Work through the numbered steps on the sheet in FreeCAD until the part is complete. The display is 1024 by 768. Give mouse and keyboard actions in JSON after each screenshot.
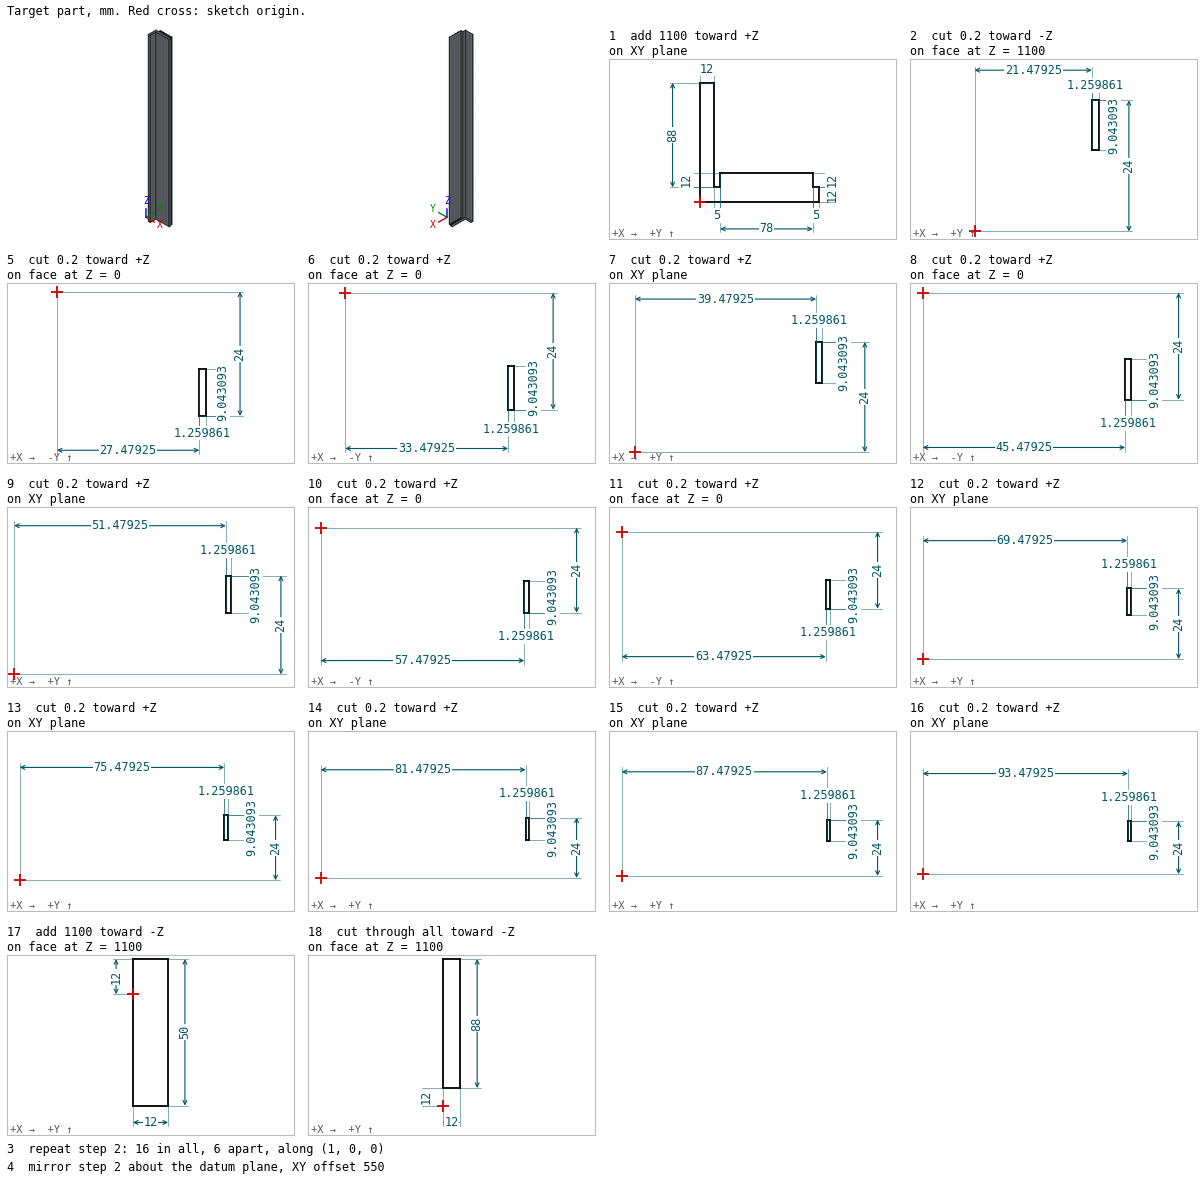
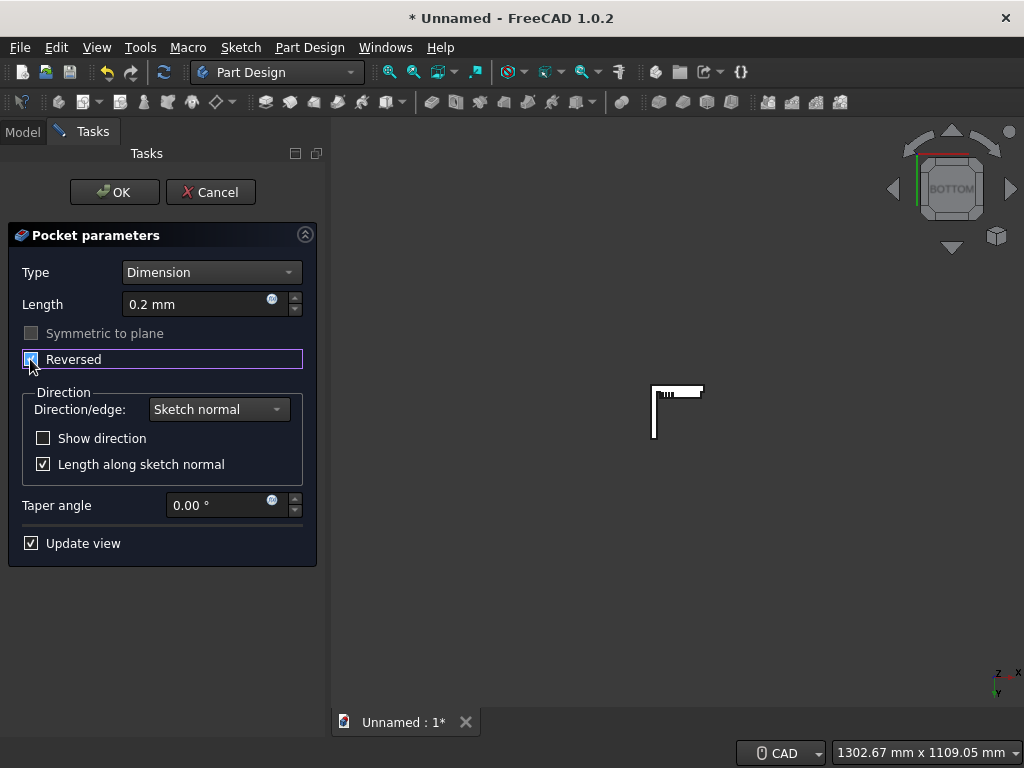
{"action": "left_click", "coordinate": [115, 192]}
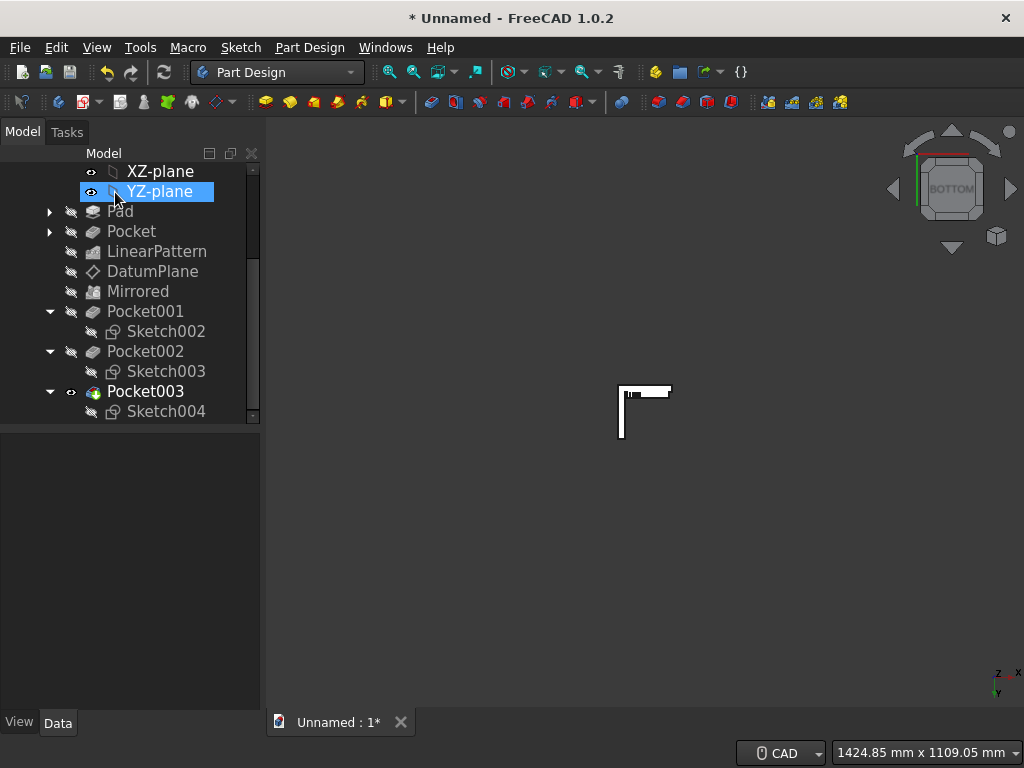
{"action": "left_click", "coordinate": [390, 72]}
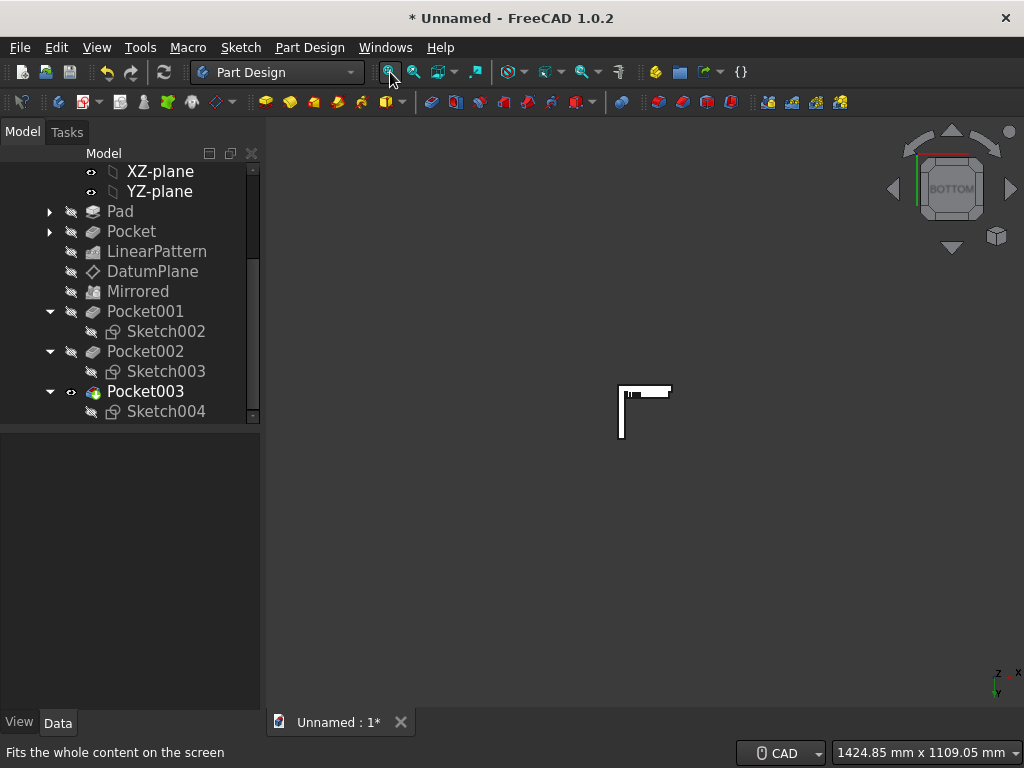
{"action": "left_click", "coordinate": [660, 388]}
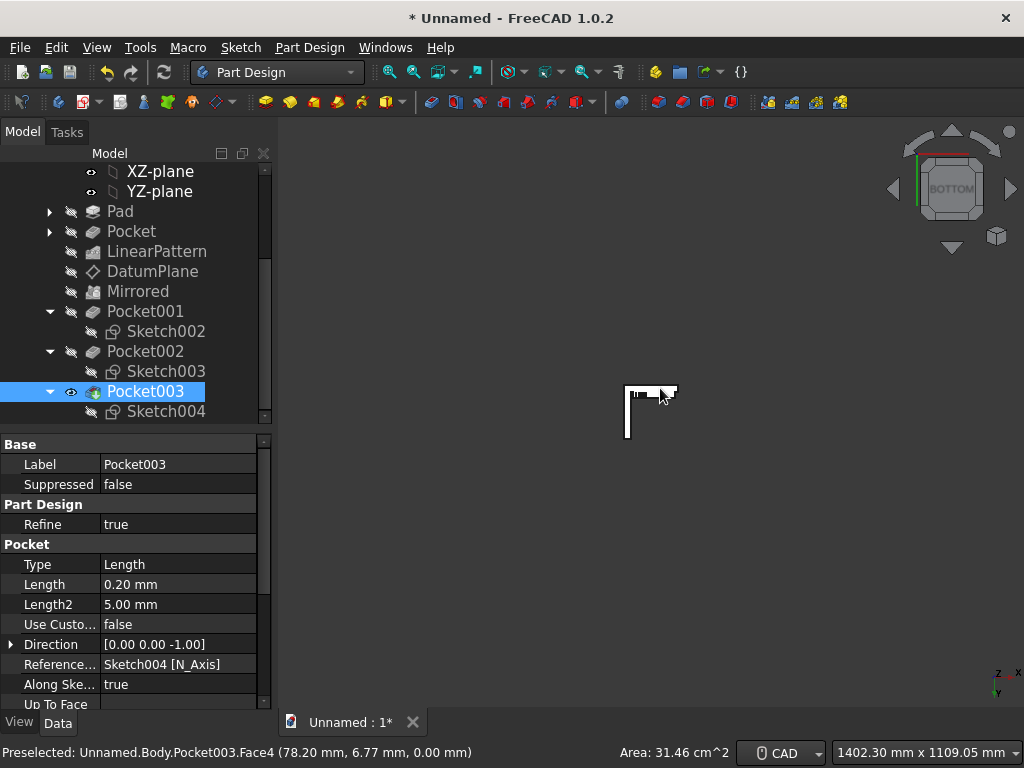
{"action": "left_click", "coordinate": [84, 102]}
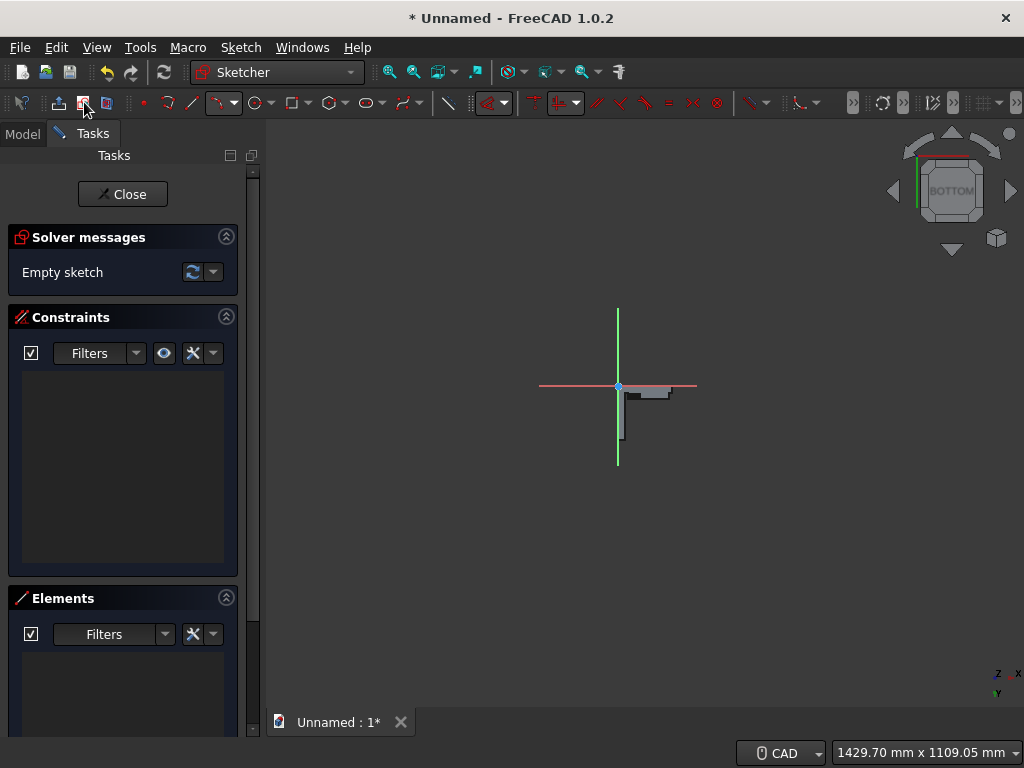
{"action": "scroll", "coordinate": [646, 396], "scroll_direction": "up", "scroll_amount": 15}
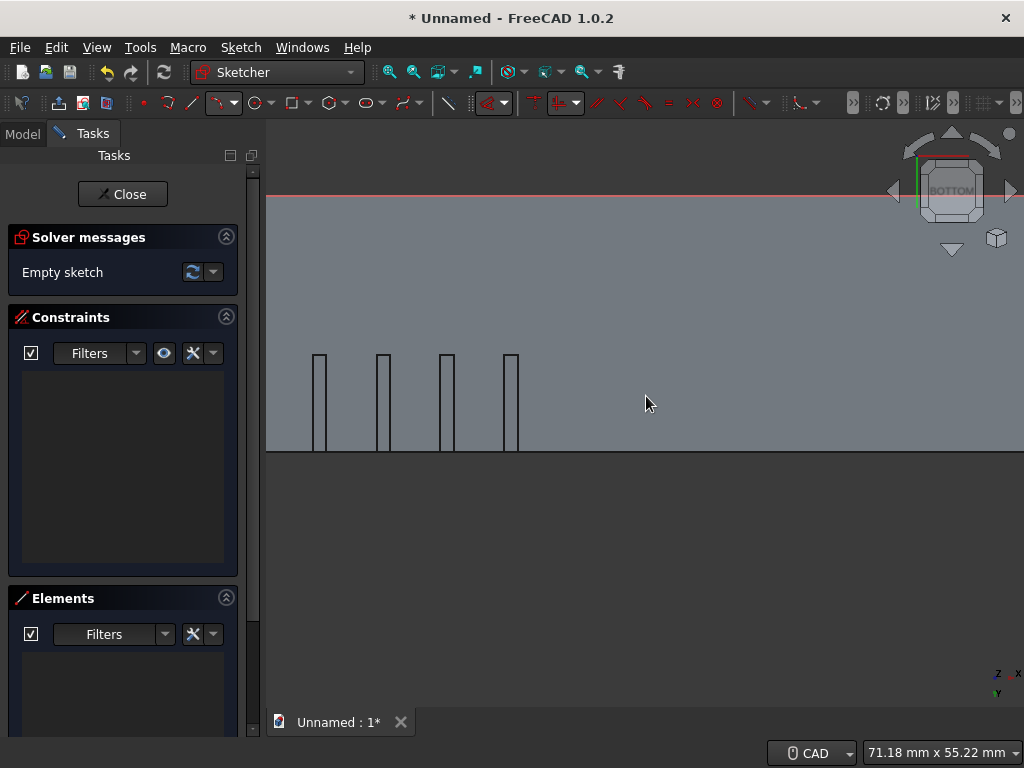
{"action": "scroll", "coordinate": [574, 400], "scroll_direction": "up", "scroll_amount": 7}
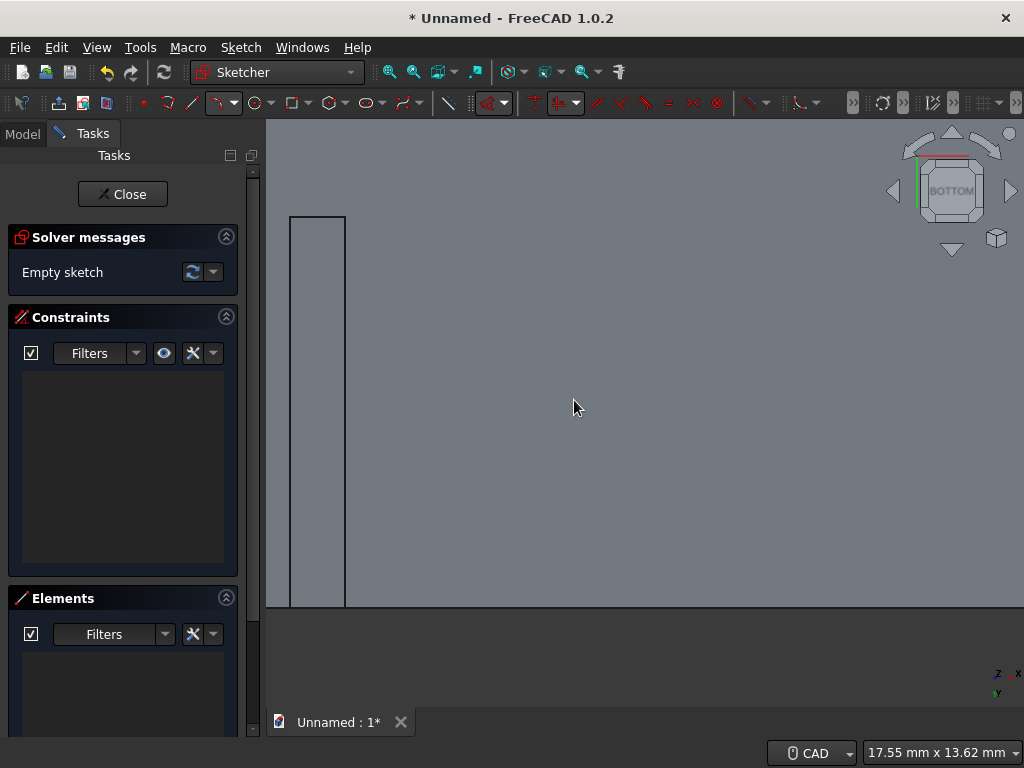
{"action": "left_click", "coordinate": [292, 104]}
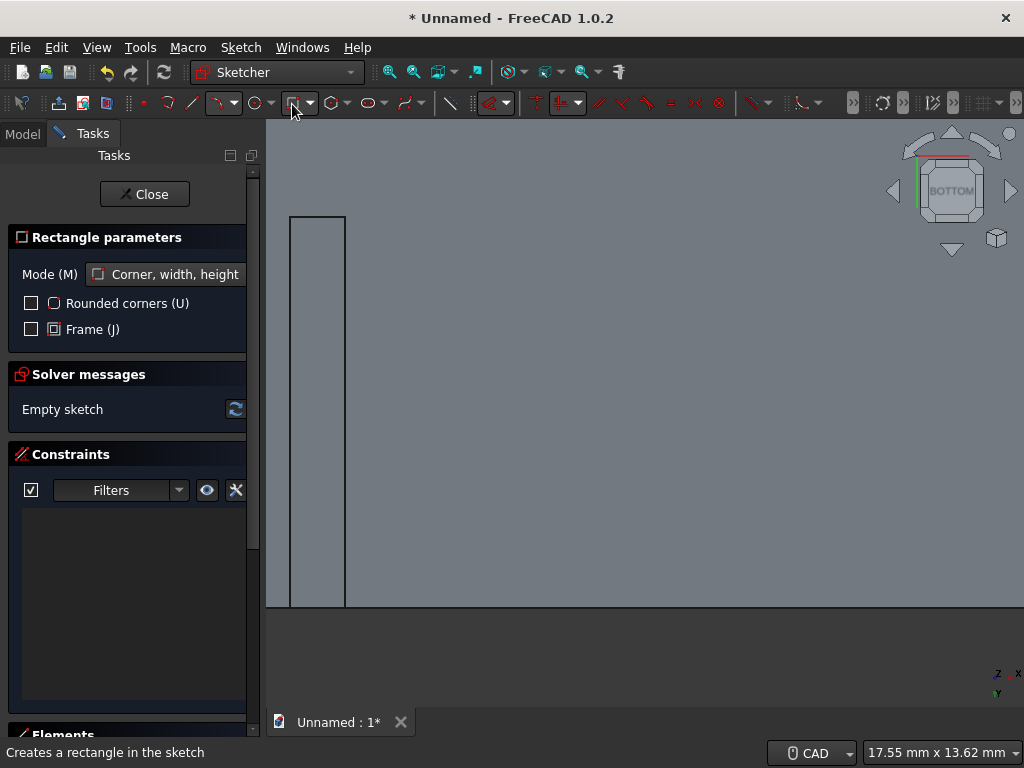
{"action": "left_click", "coordinate": [549, 217]}
{"action": "mouse_move", "coordinate": [604, 608]}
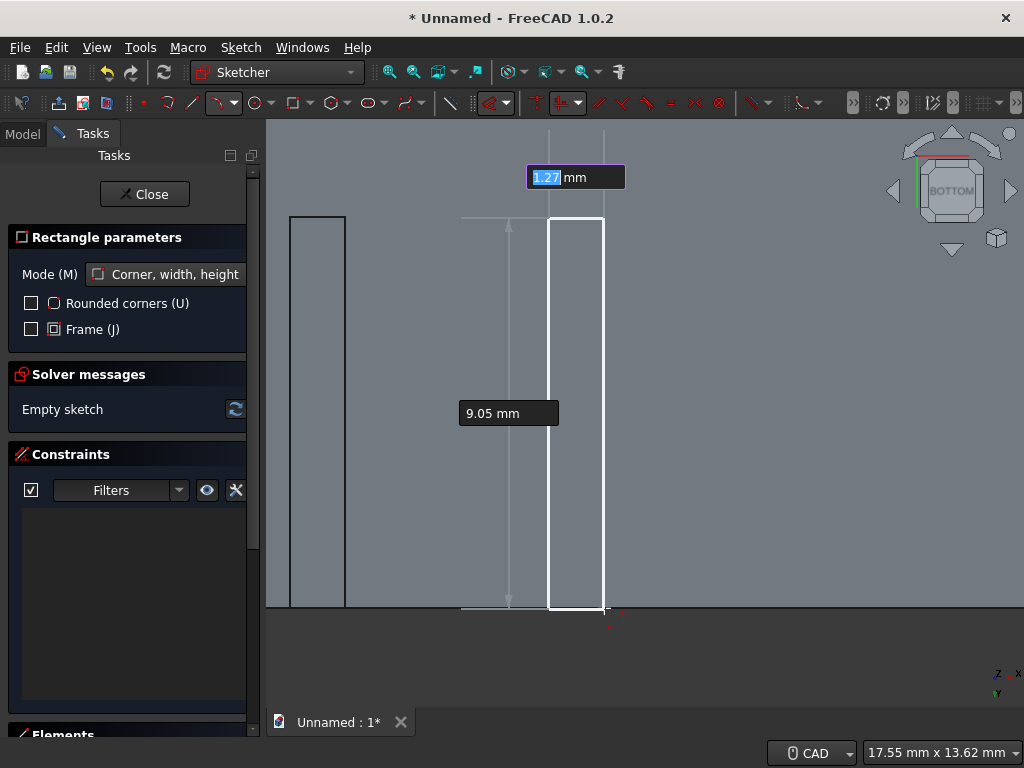
{"action": "type", "text": "1.259861"}
{"action": "key", "text": "Tab"}
{"action": "type", "text": "9.043093"}
{"action": "key", "text": "Return"}
{"action": "key", "text": "Escape"}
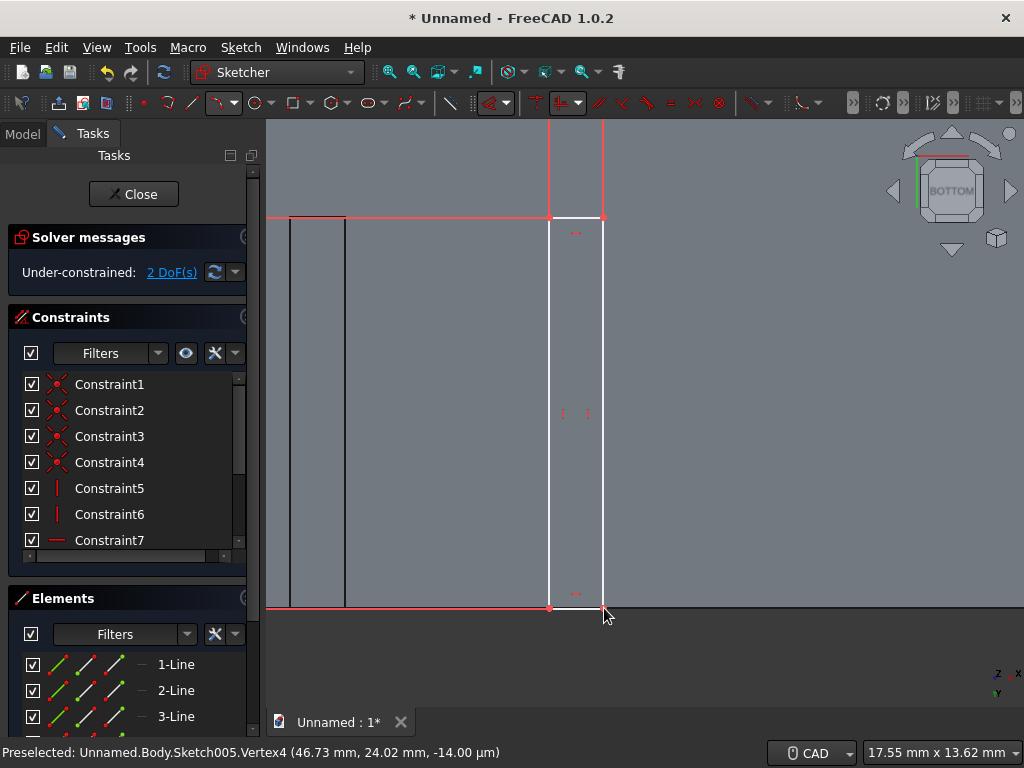
{"action": "left_click", "coordinate": [549, 609]}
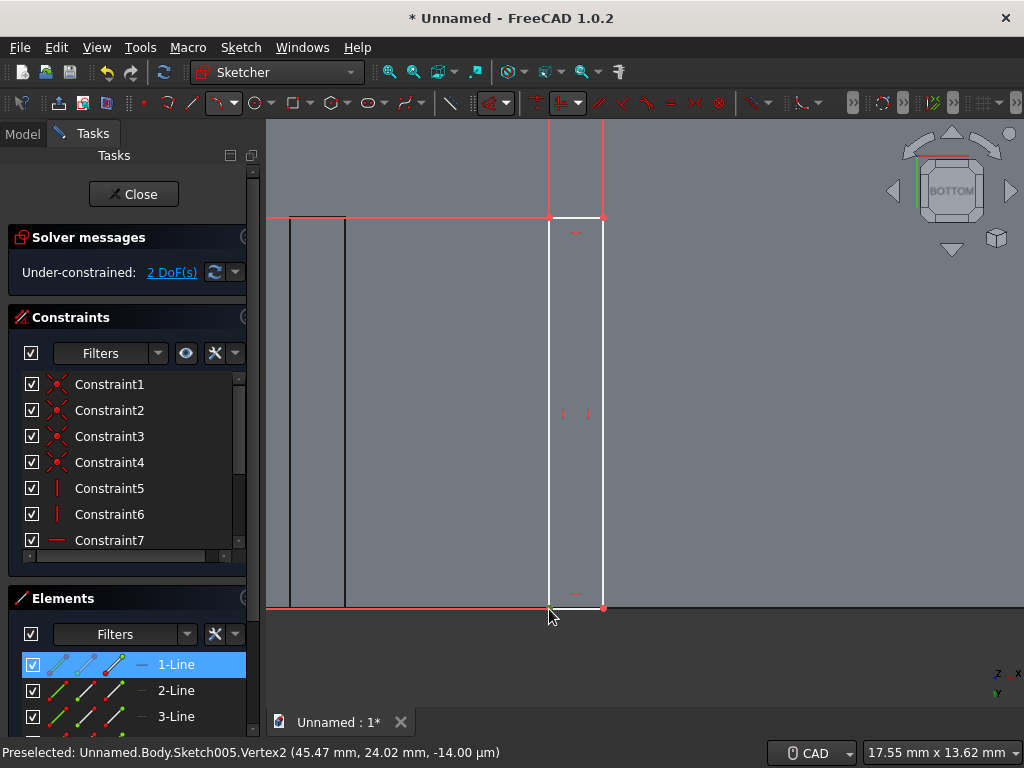
{"action": "left_click", "coordinate": [508, 104]}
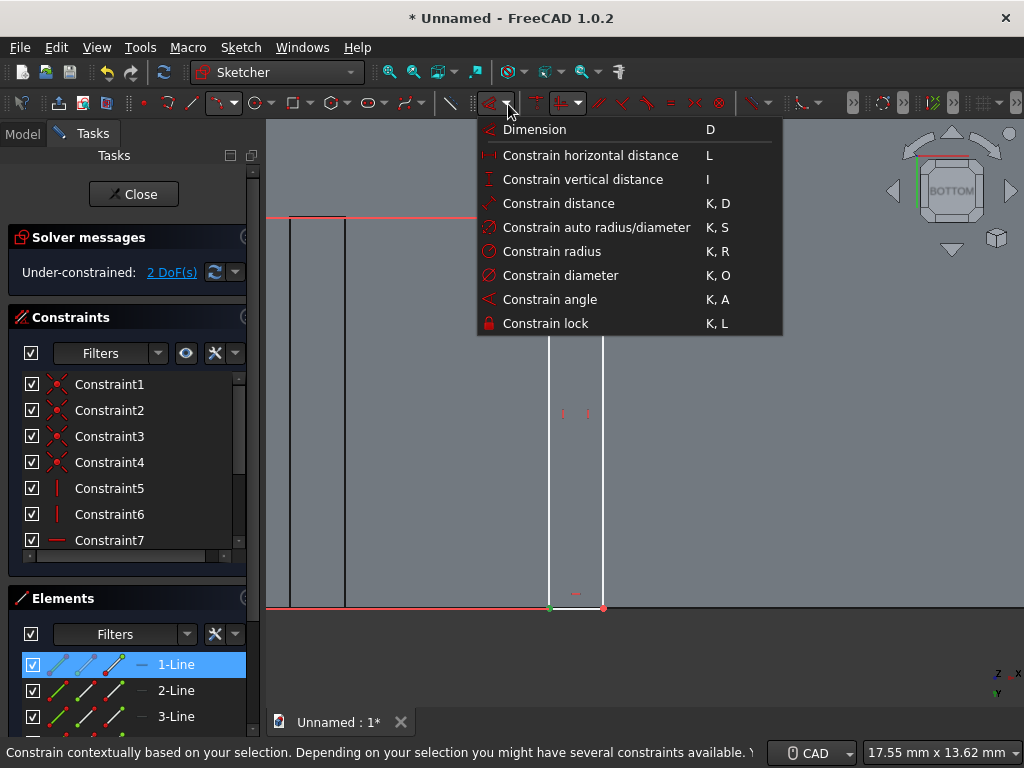
{"action": "left_click", "coordinate": [630, 179]}